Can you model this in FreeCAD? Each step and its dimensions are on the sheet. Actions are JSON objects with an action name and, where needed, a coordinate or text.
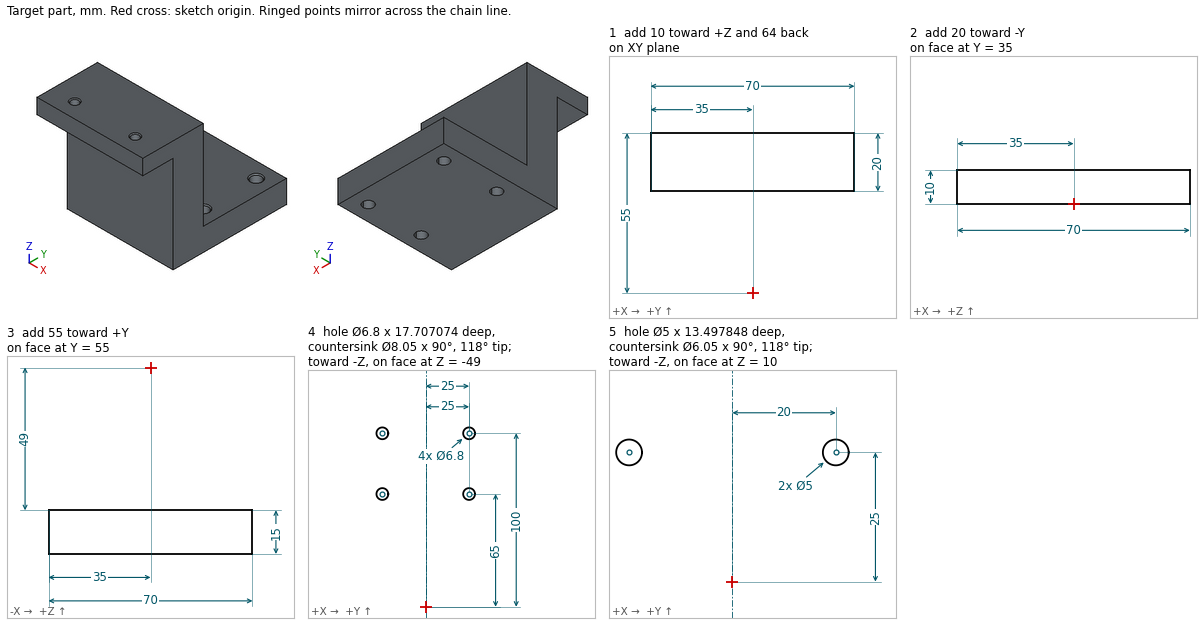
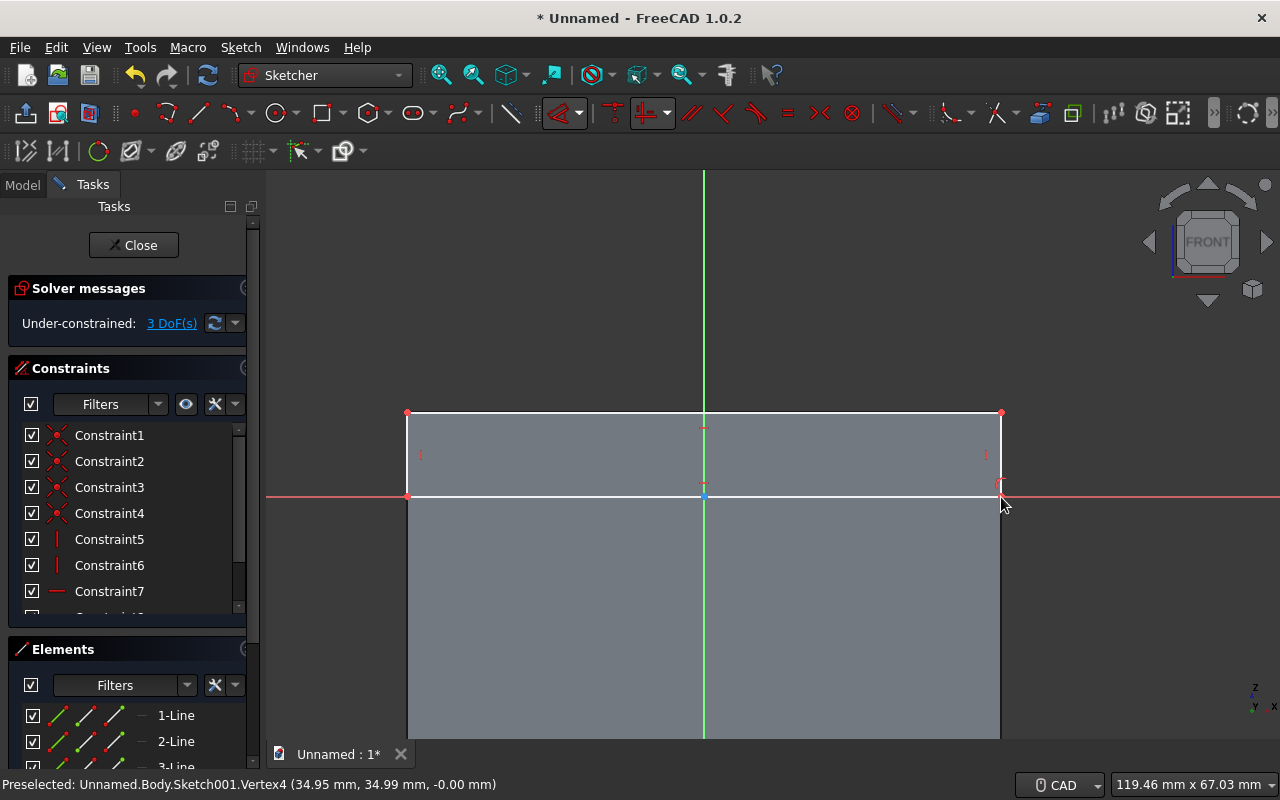
{"action": "left_click", "coordinate": [407, 438]}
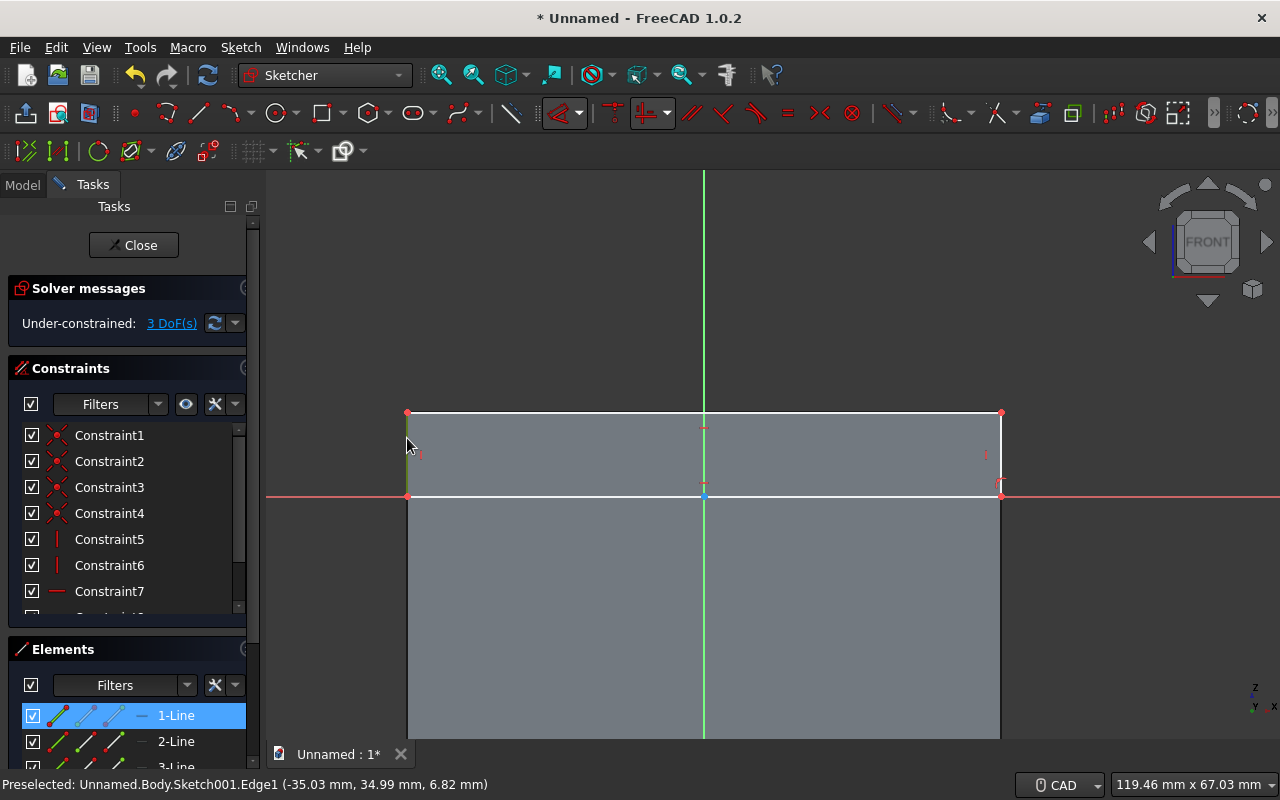
{"action": "key", "text": "i"}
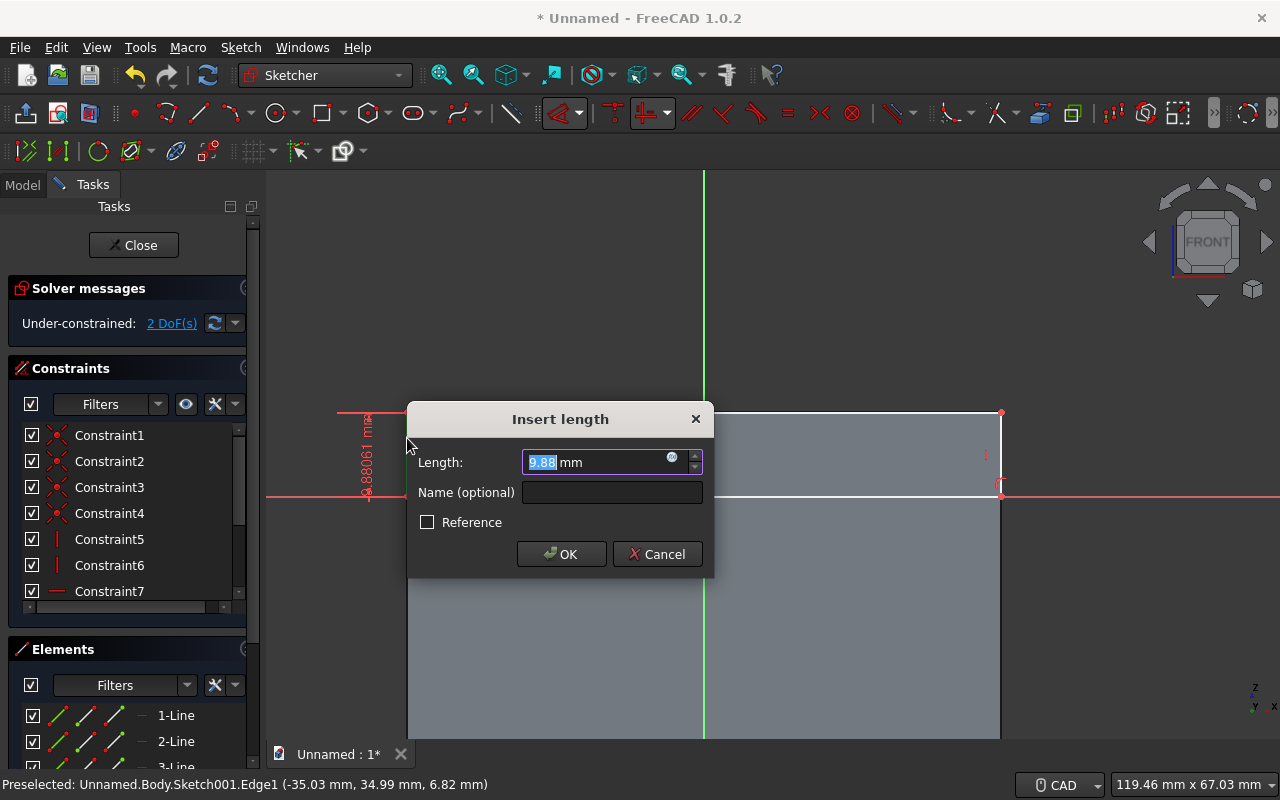
{"action": "type", "text": "10"}
{"action": "key", "text": "Return"}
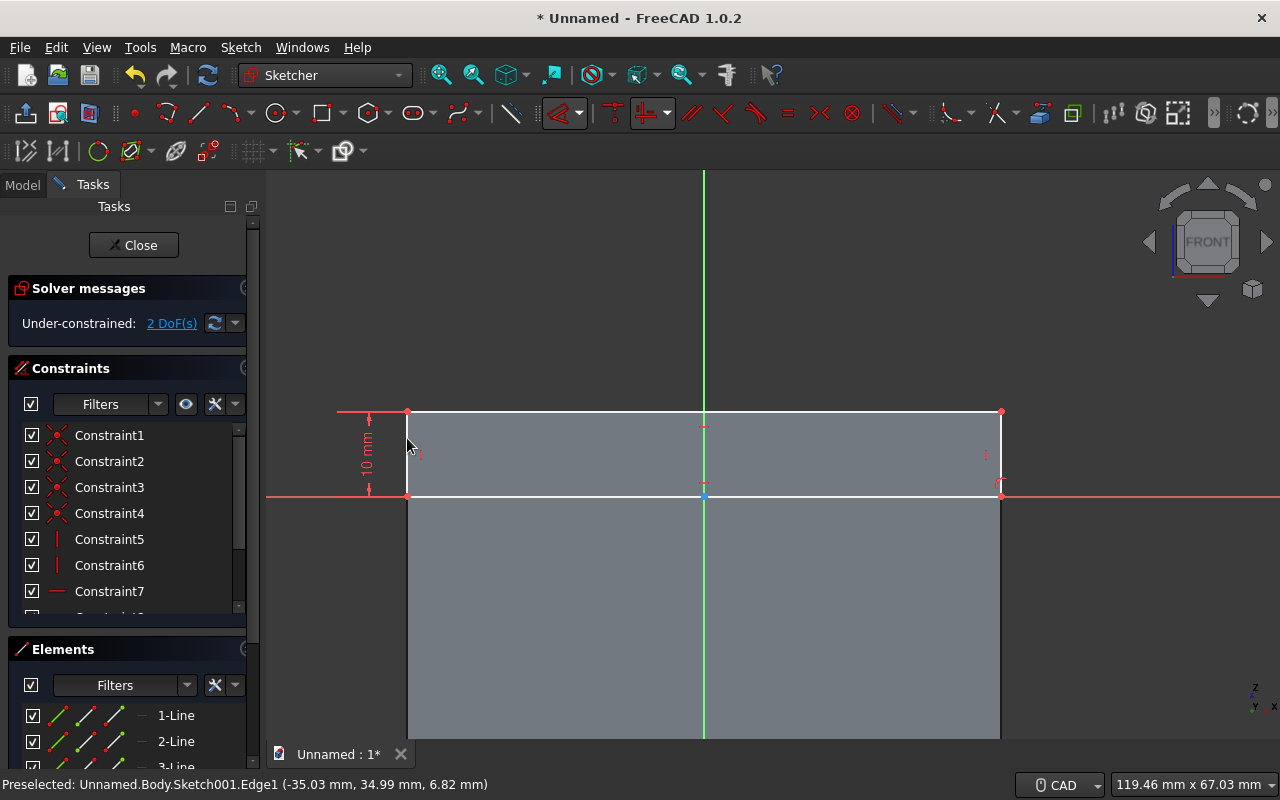
{"action": "left_click", "coordinate": [585, 497]}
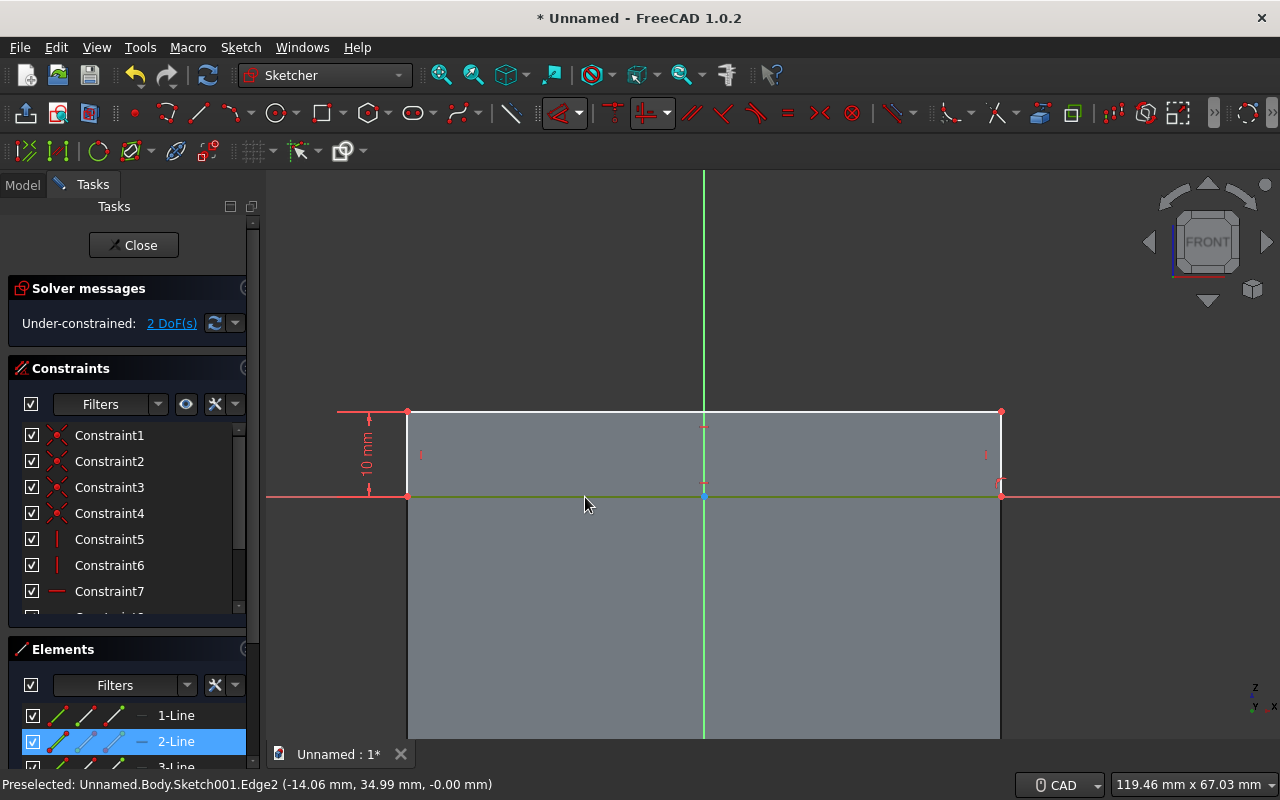
{"action": "left_click", "coordinate": [582, 114]}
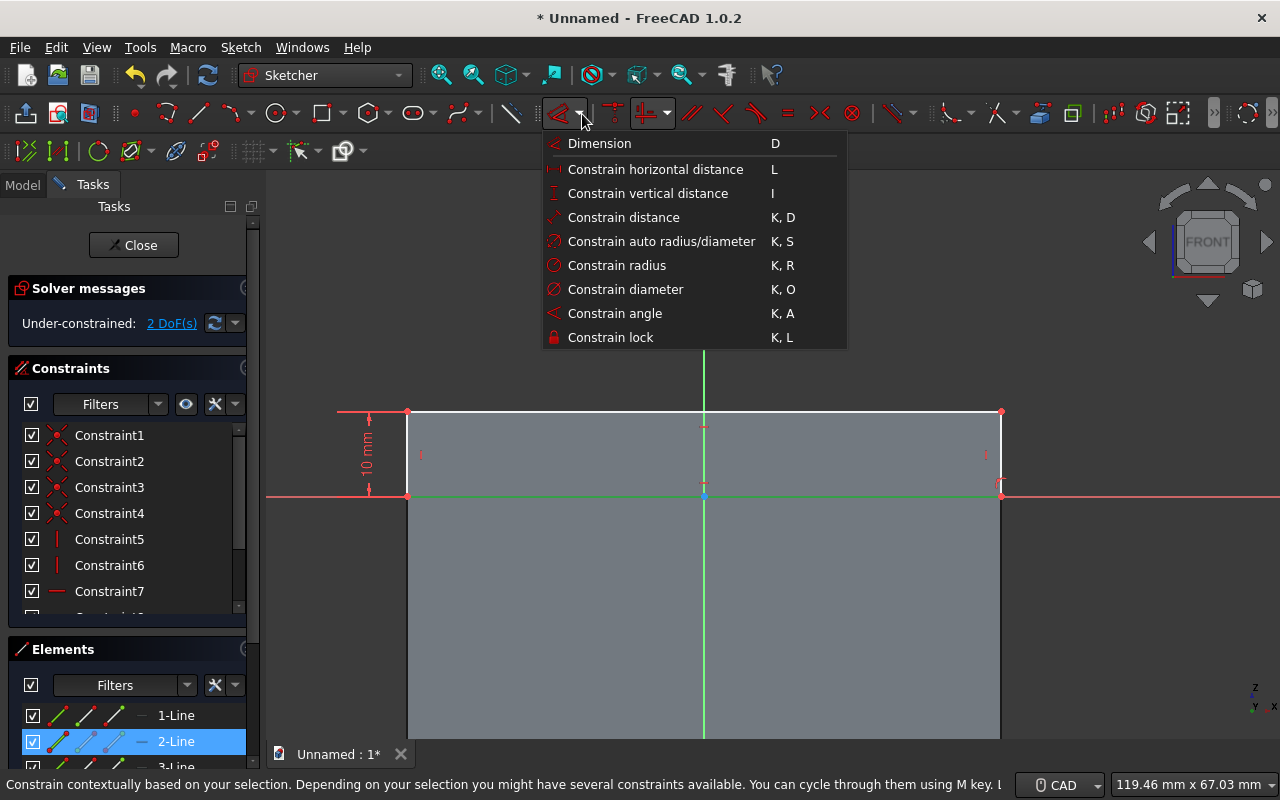
{"action": "left_click", "coordinate": [695, 169]}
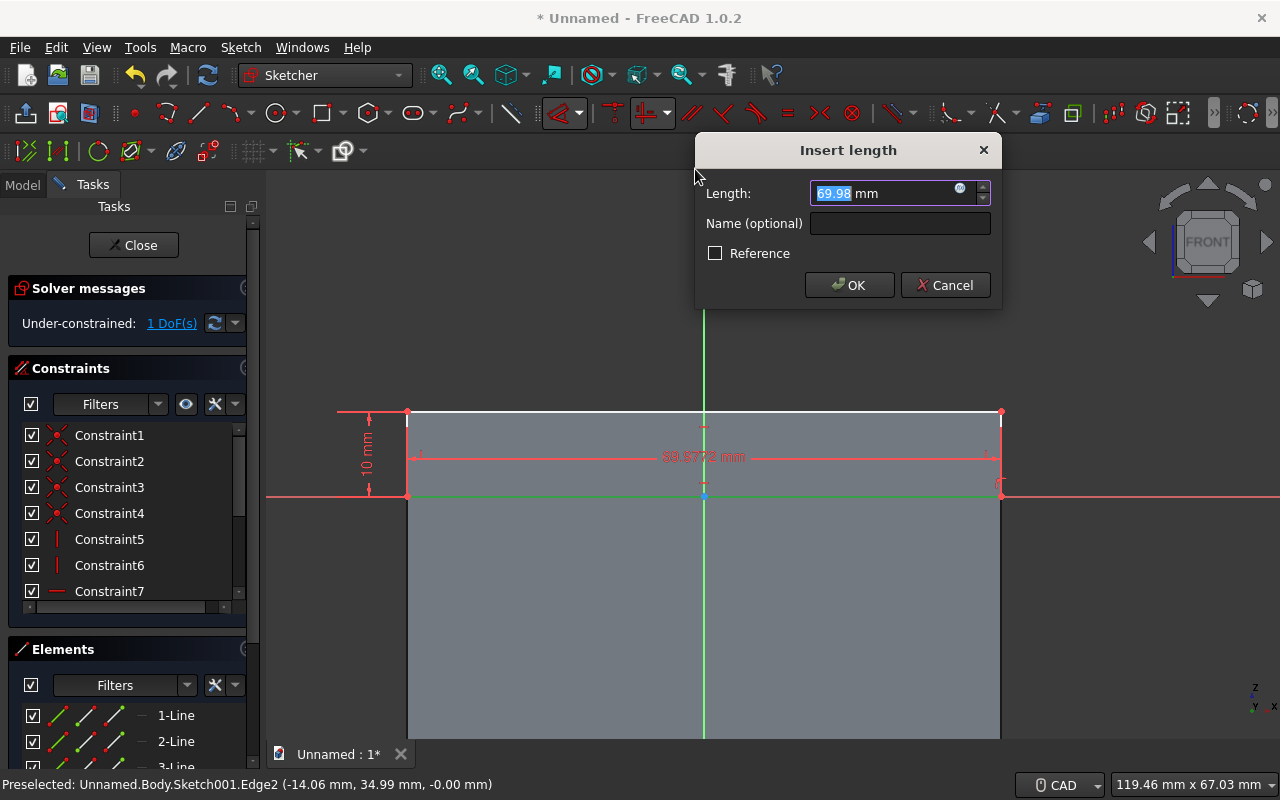
{"action": "type", "text": "70"}
{"action": "key", "text": "Return"}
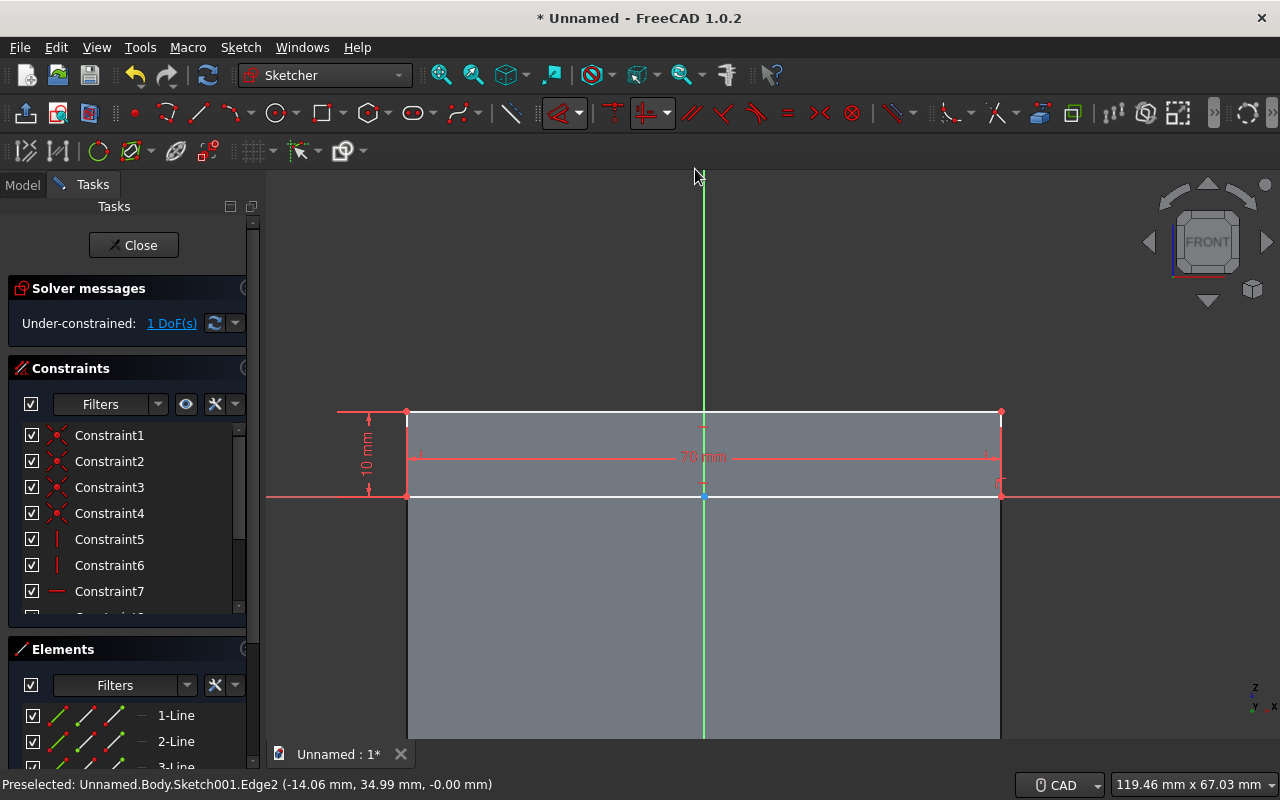
{"action": "left_click", "coordinate": [407, 412]}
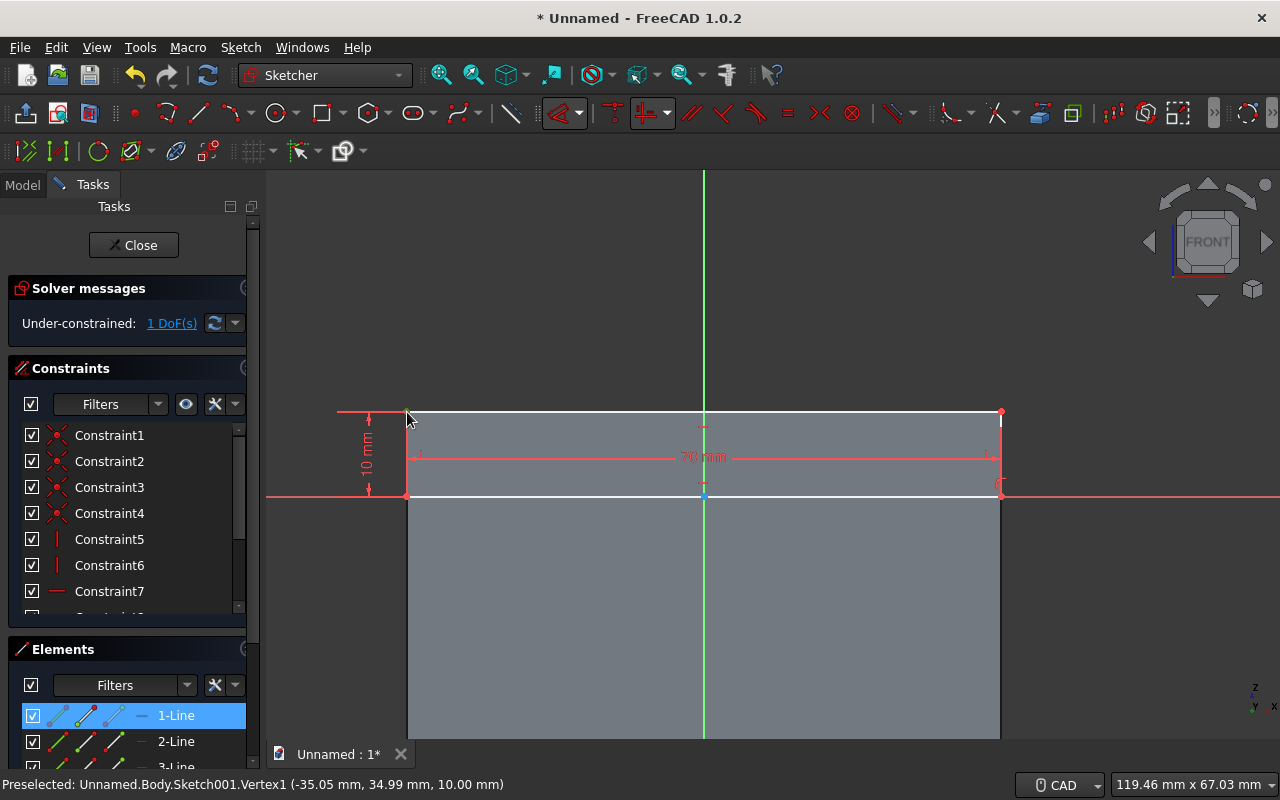
{"action": "key", "text": "l"}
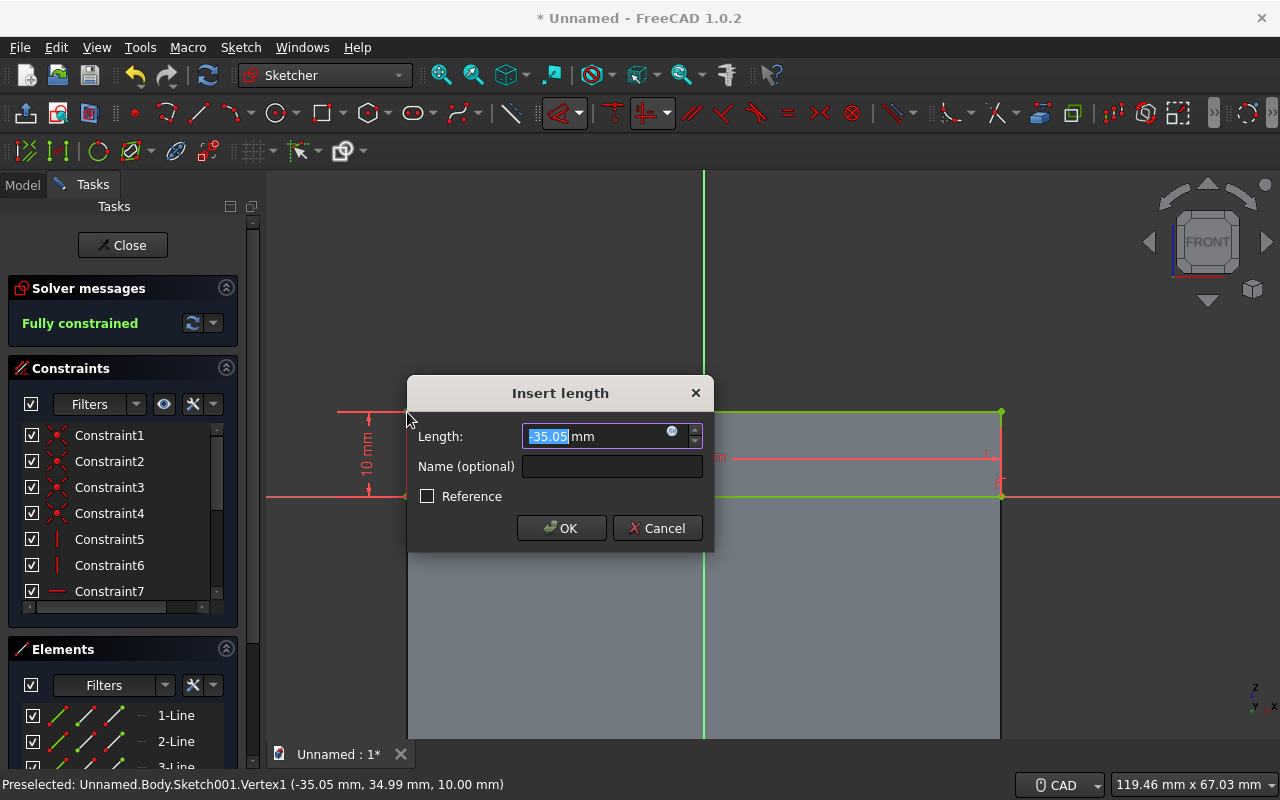
{"action": "type", "text": "-35"}
{"action": "key", "text": "Return"}